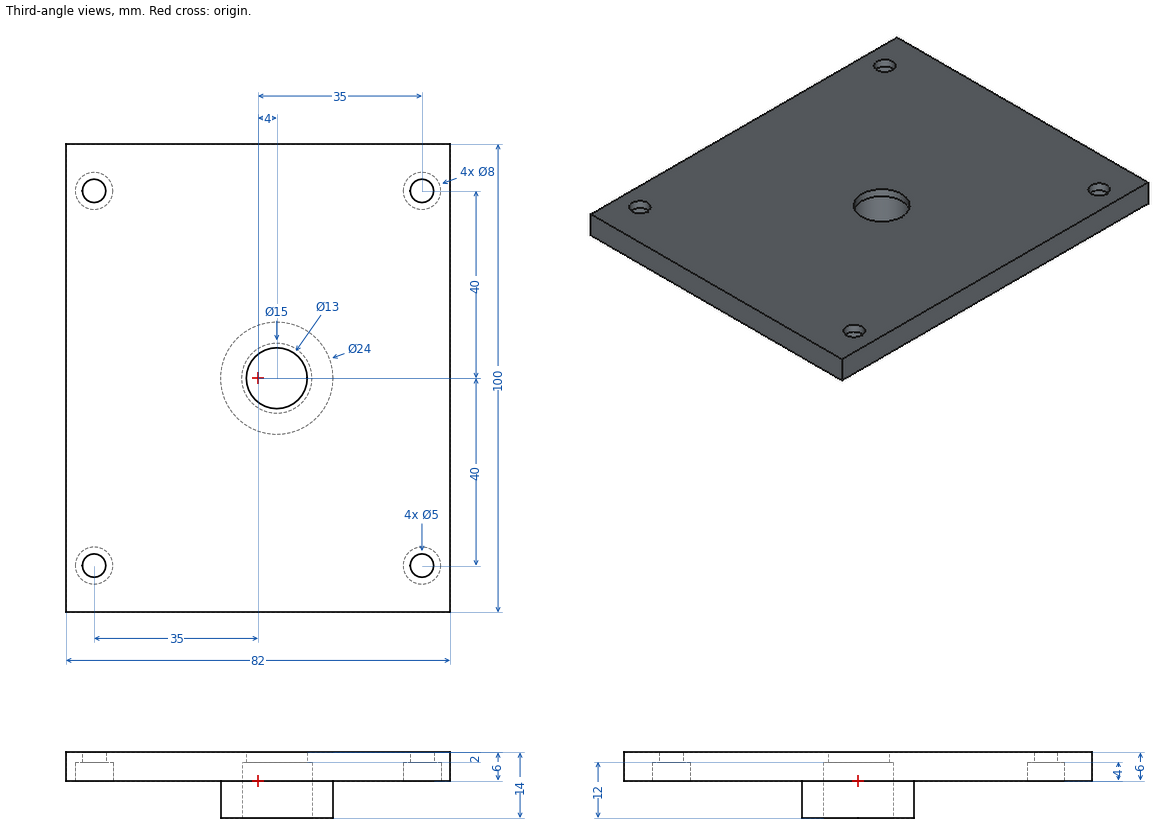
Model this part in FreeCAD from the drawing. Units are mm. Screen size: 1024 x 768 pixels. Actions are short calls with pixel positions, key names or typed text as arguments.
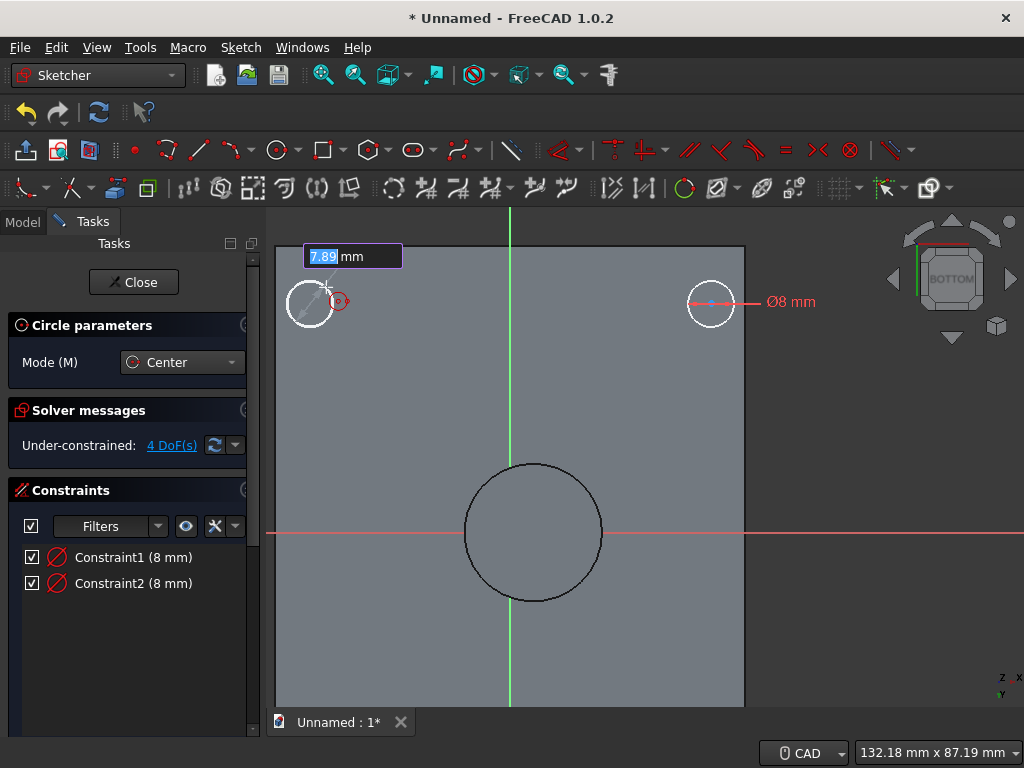
text(8)
key(Return)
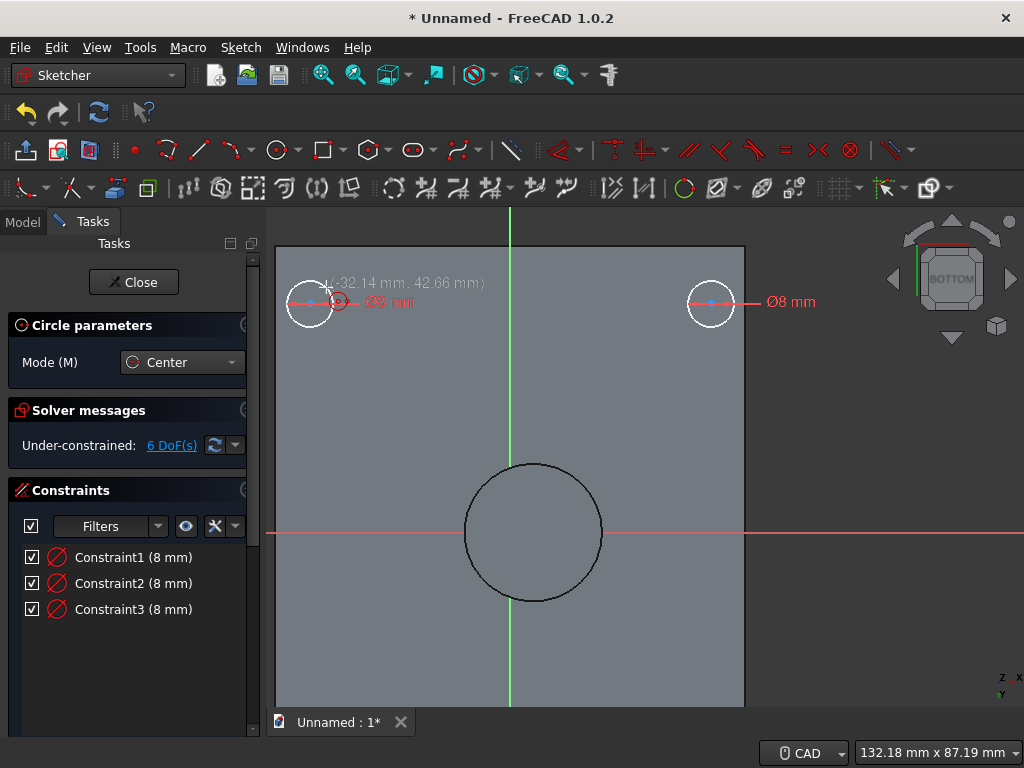
scroll(711, 303, down, 2)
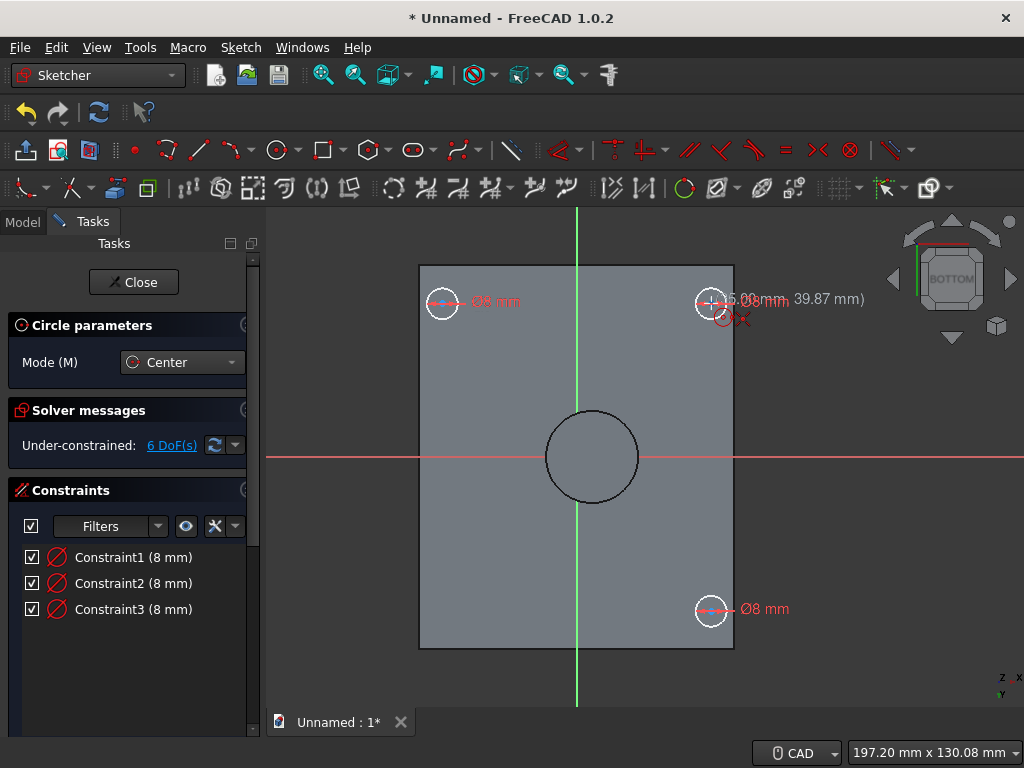
scroll(442, 611, up, 2)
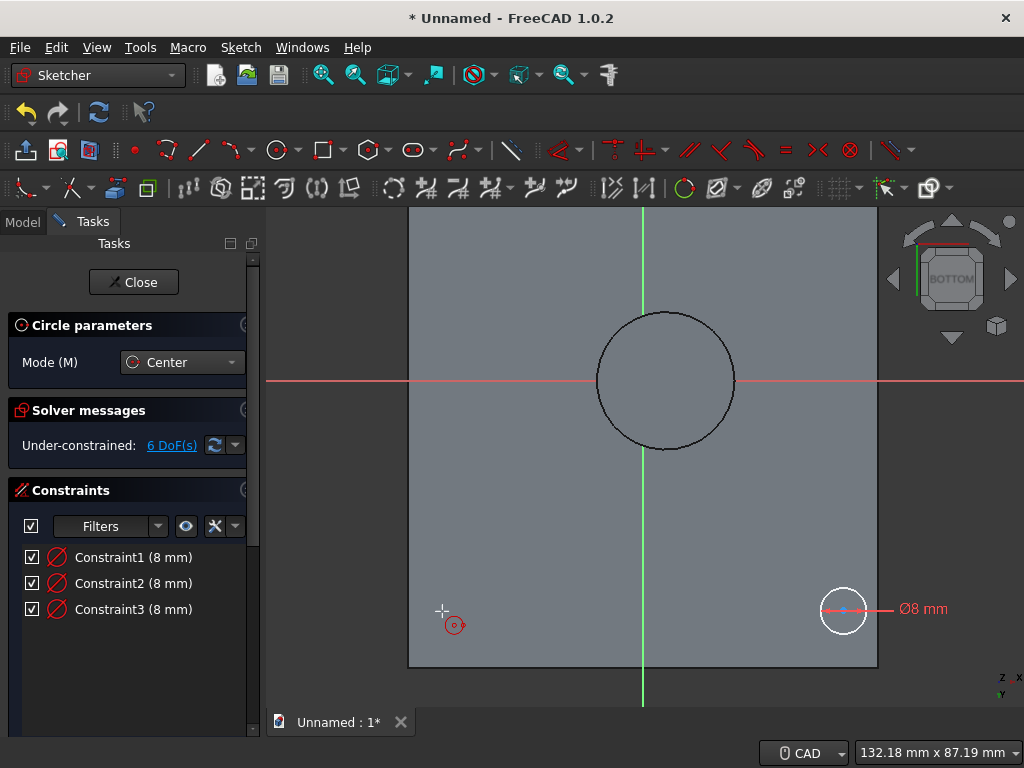
click(442, 610)
move(458, 594)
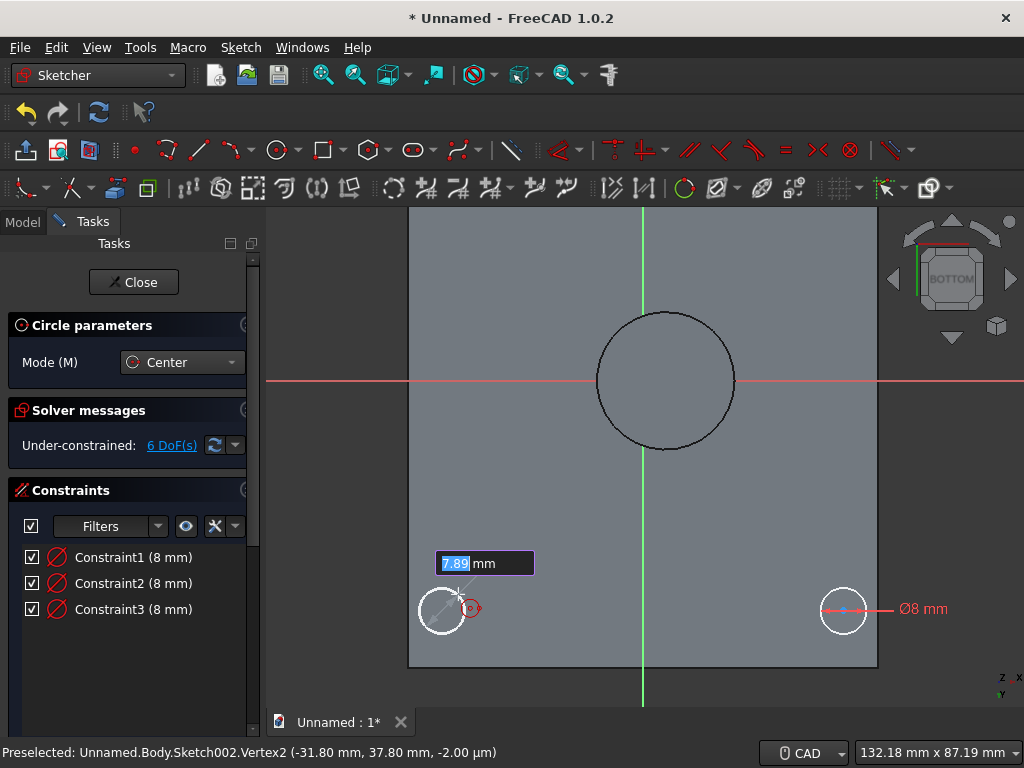
text(8)
key(Return)
key(Escape)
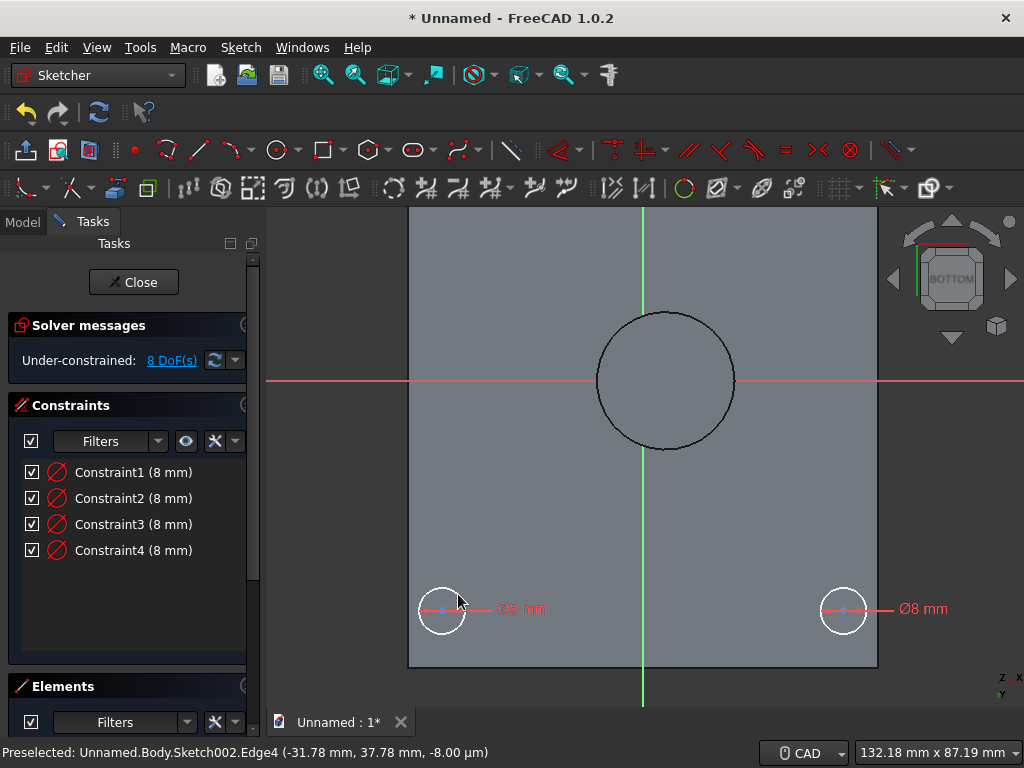
click(844, 611)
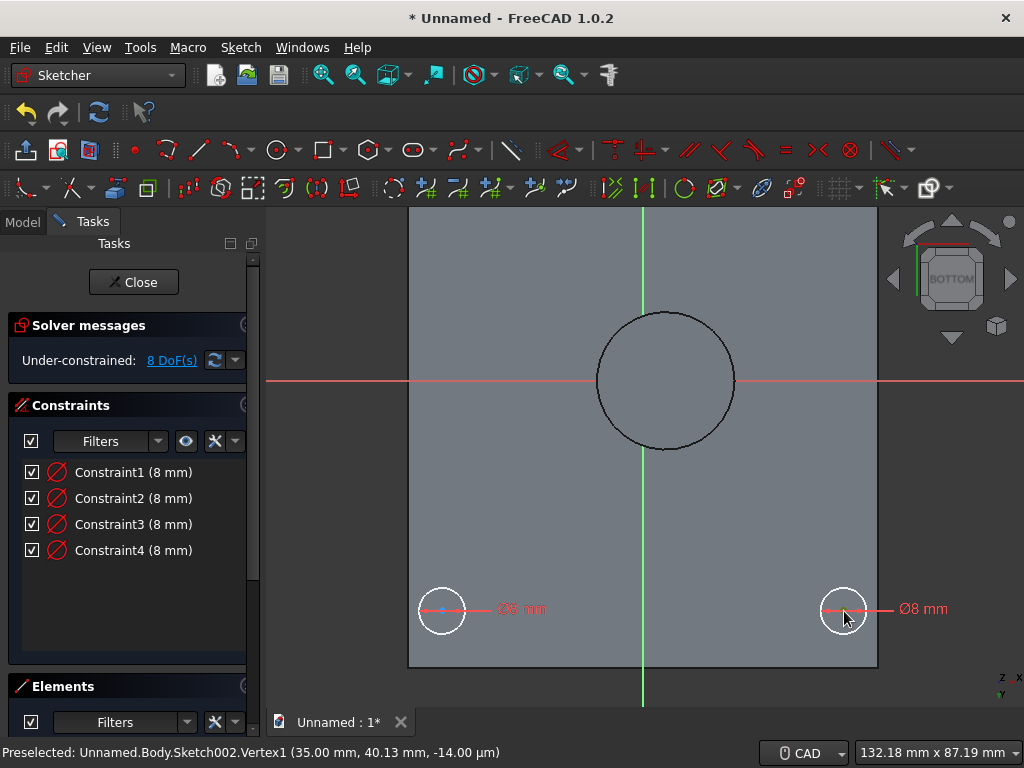
scroll(442, 612, down, 2)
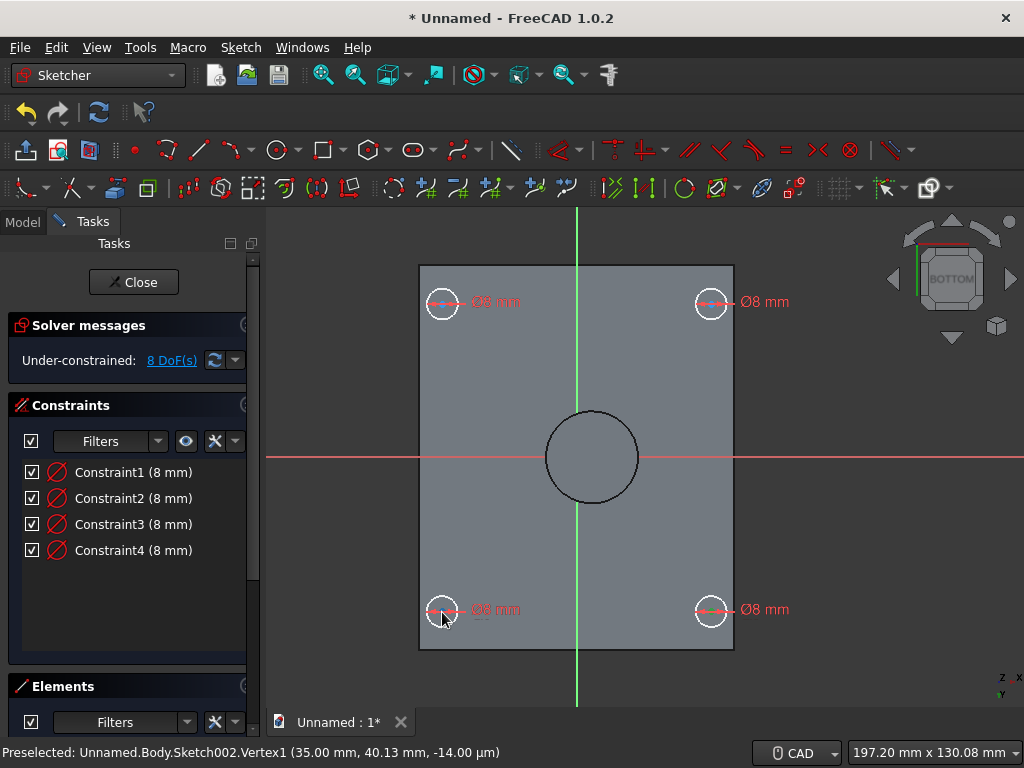
click(711, 304)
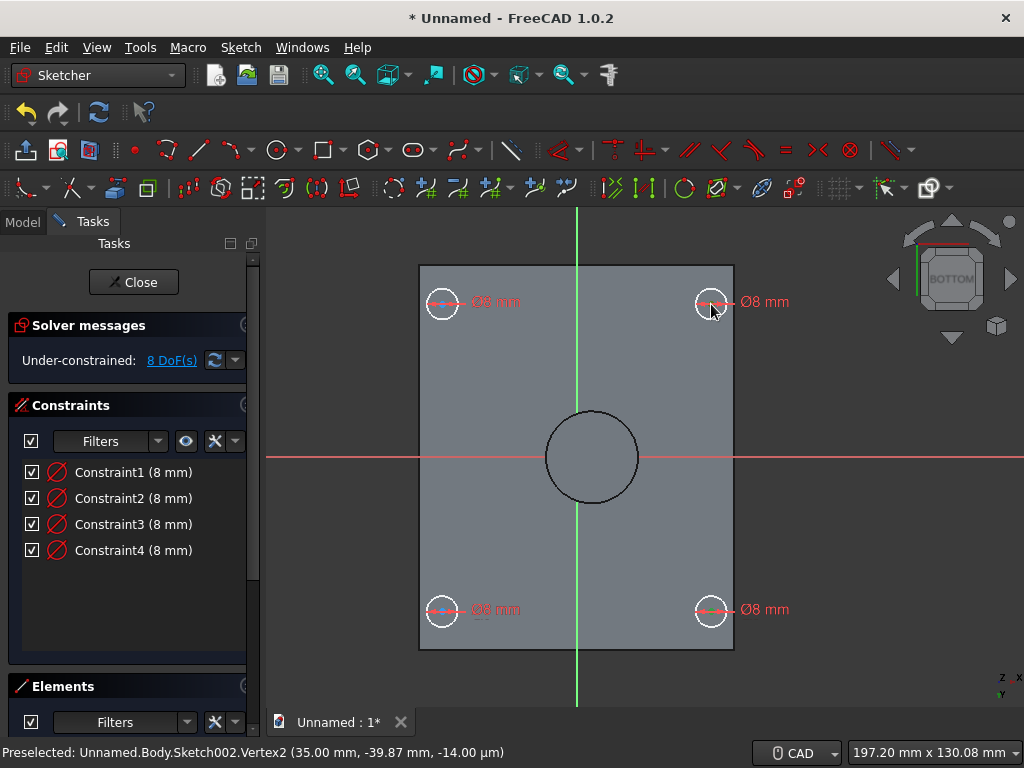
key(v)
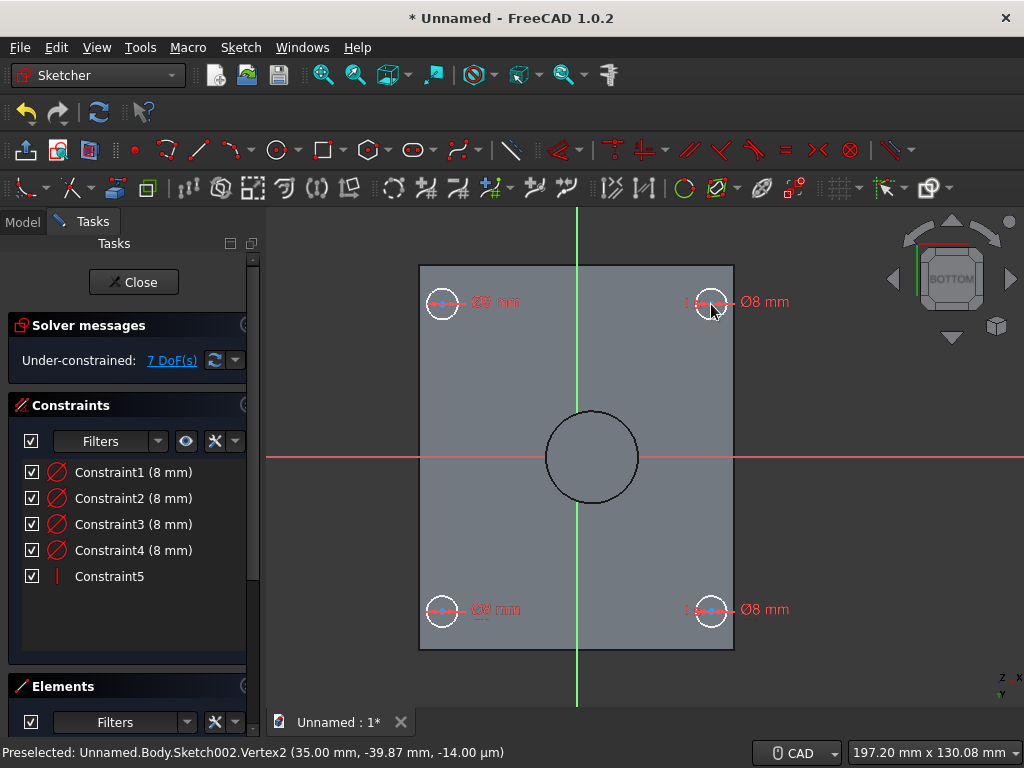
click(711, 304)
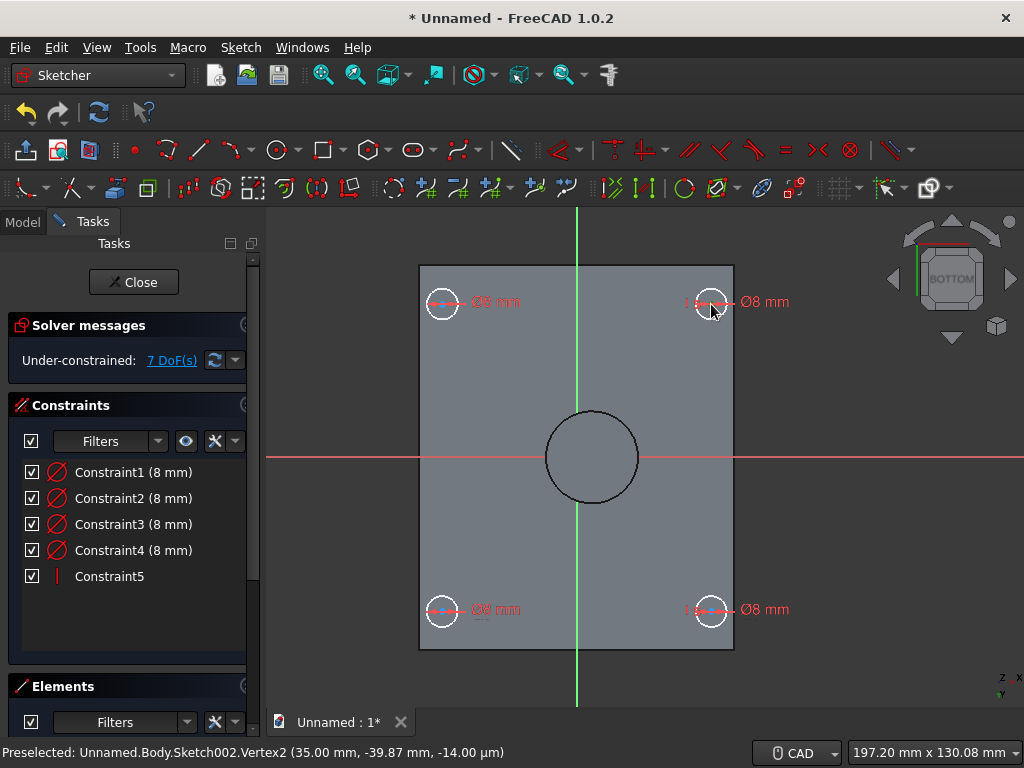
click(442, 304)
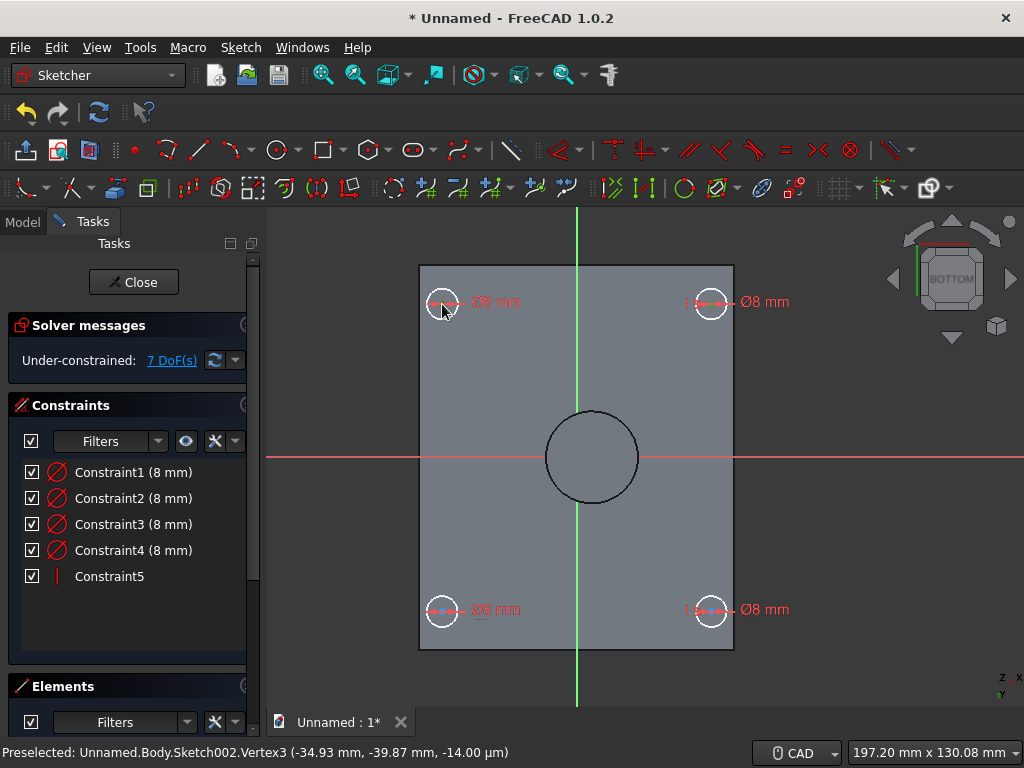
key(h)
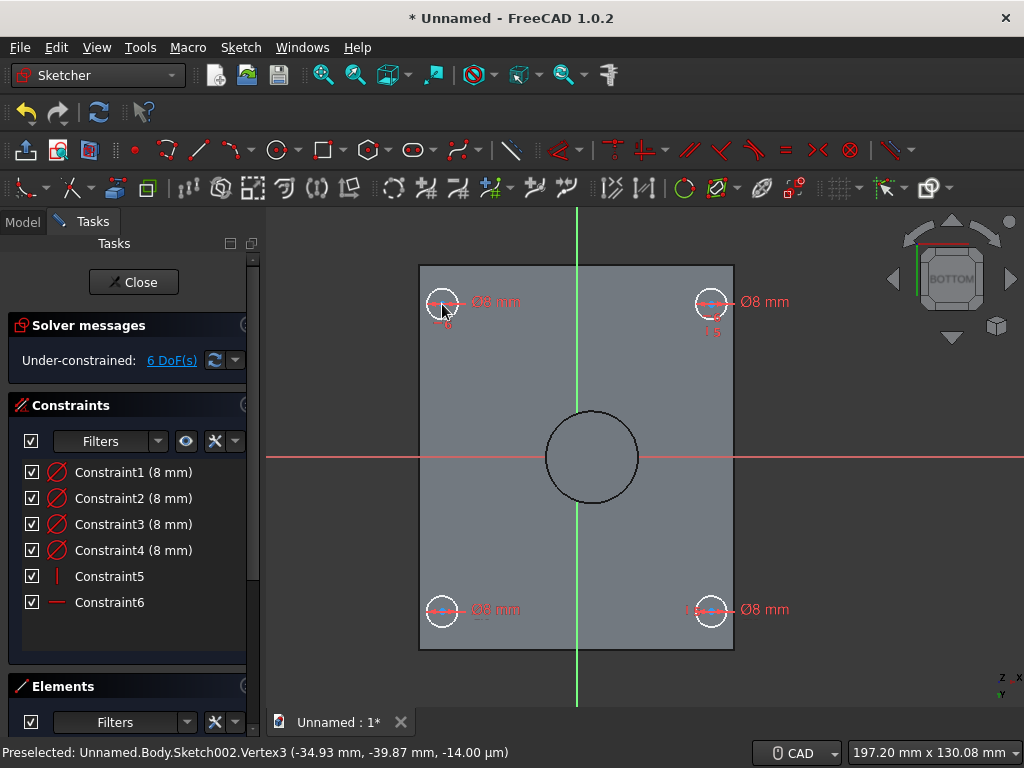
click(442, 304)